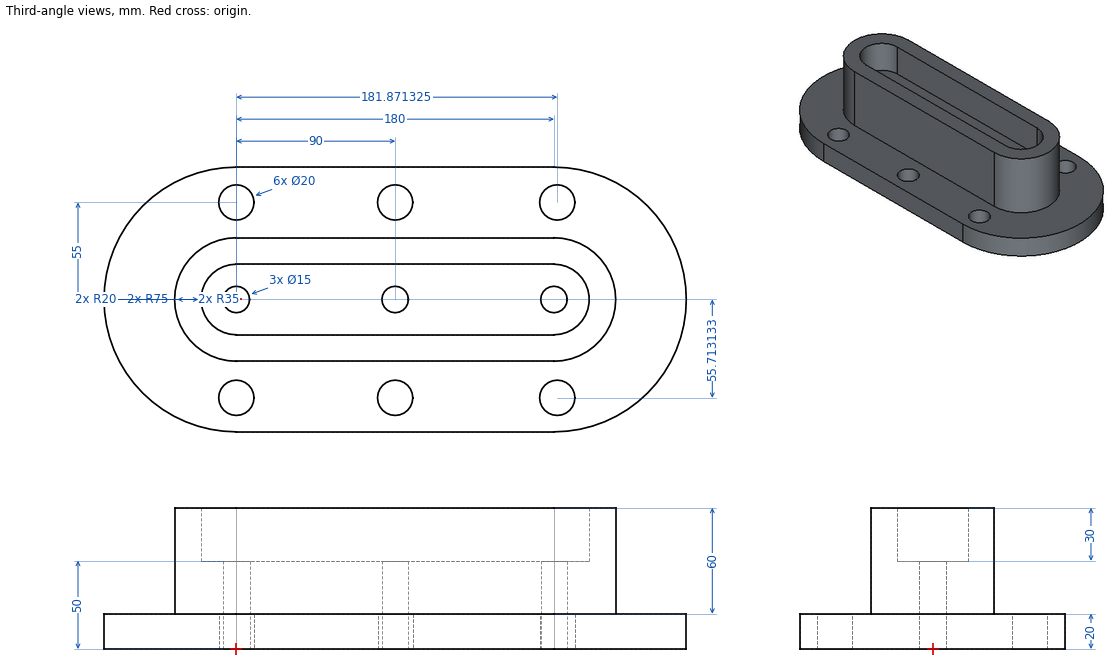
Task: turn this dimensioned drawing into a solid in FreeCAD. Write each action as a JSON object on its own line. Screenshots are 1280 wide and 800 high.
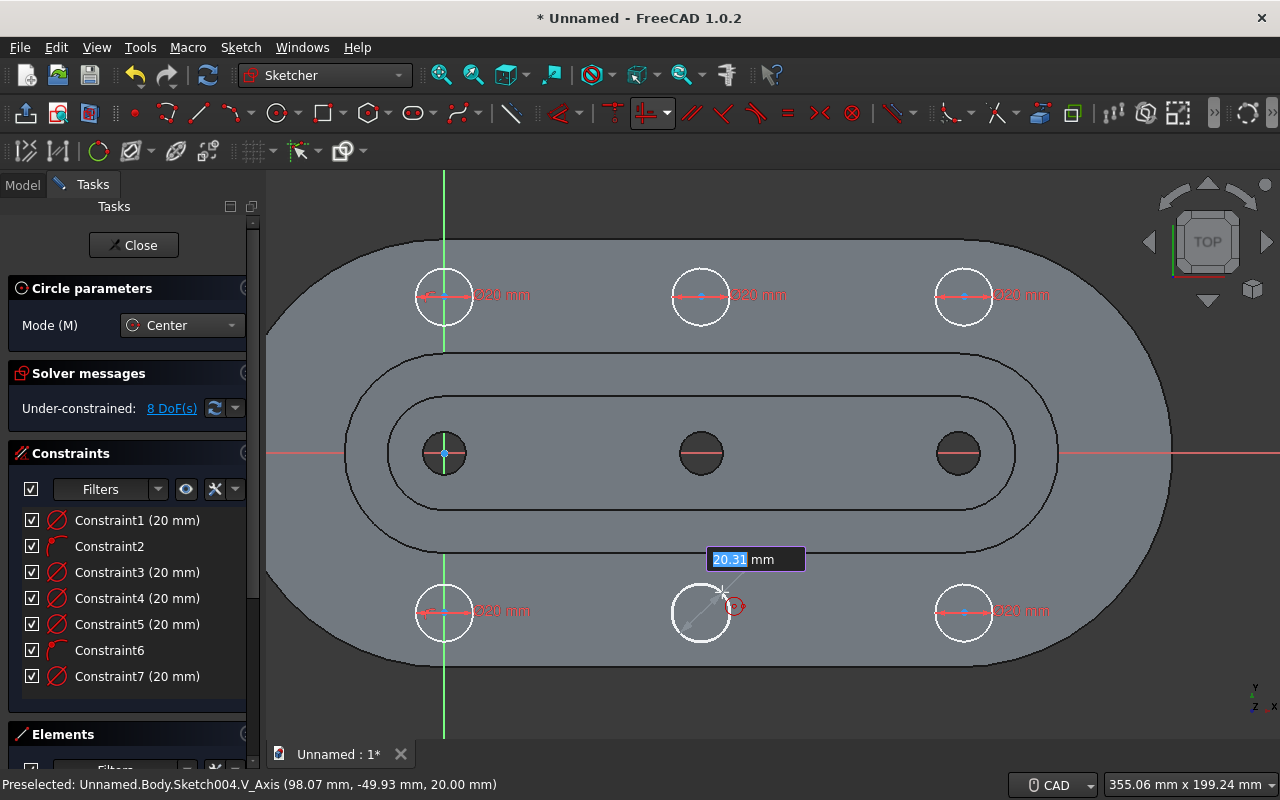
{"action": "type", "text": "20"}
{"action": "key", "text": "Return"}
{"action": "key", "text": "Escape"}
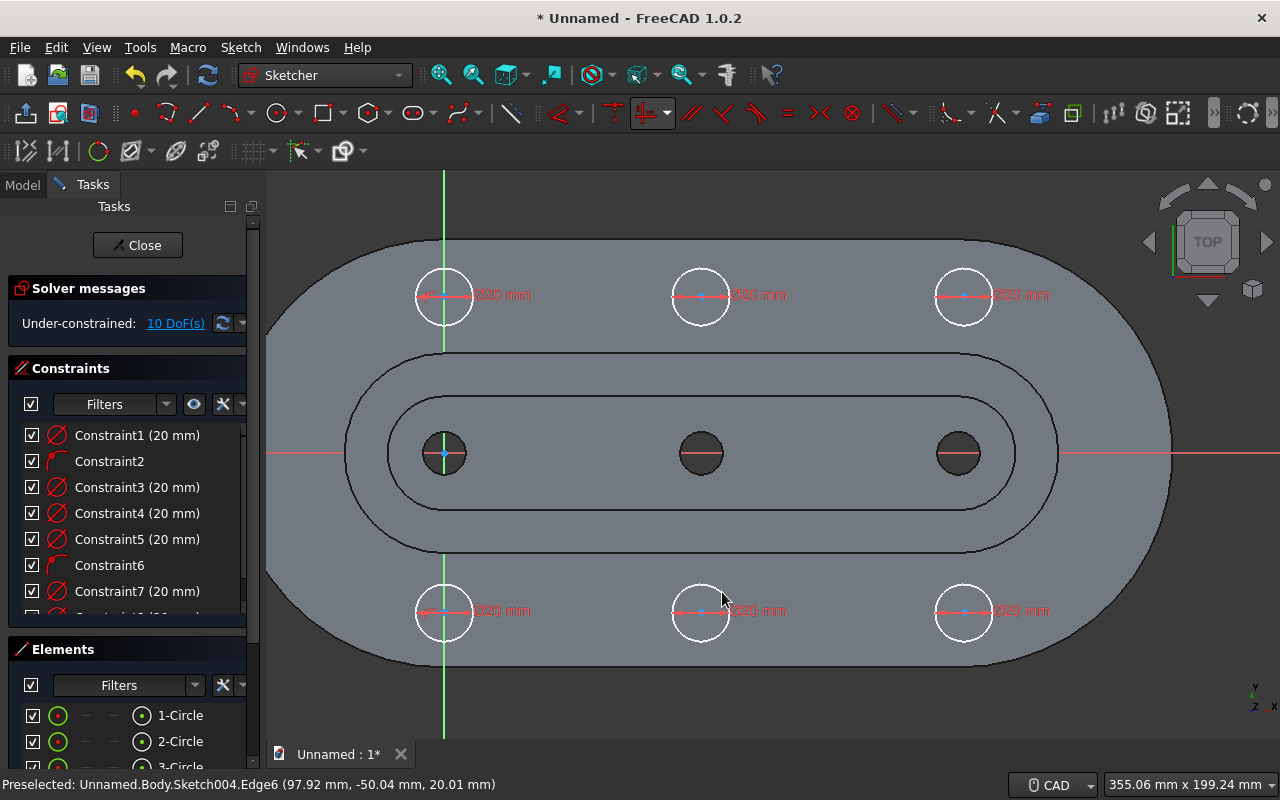
{"action": "left_click", "coordinate": [558, 114]}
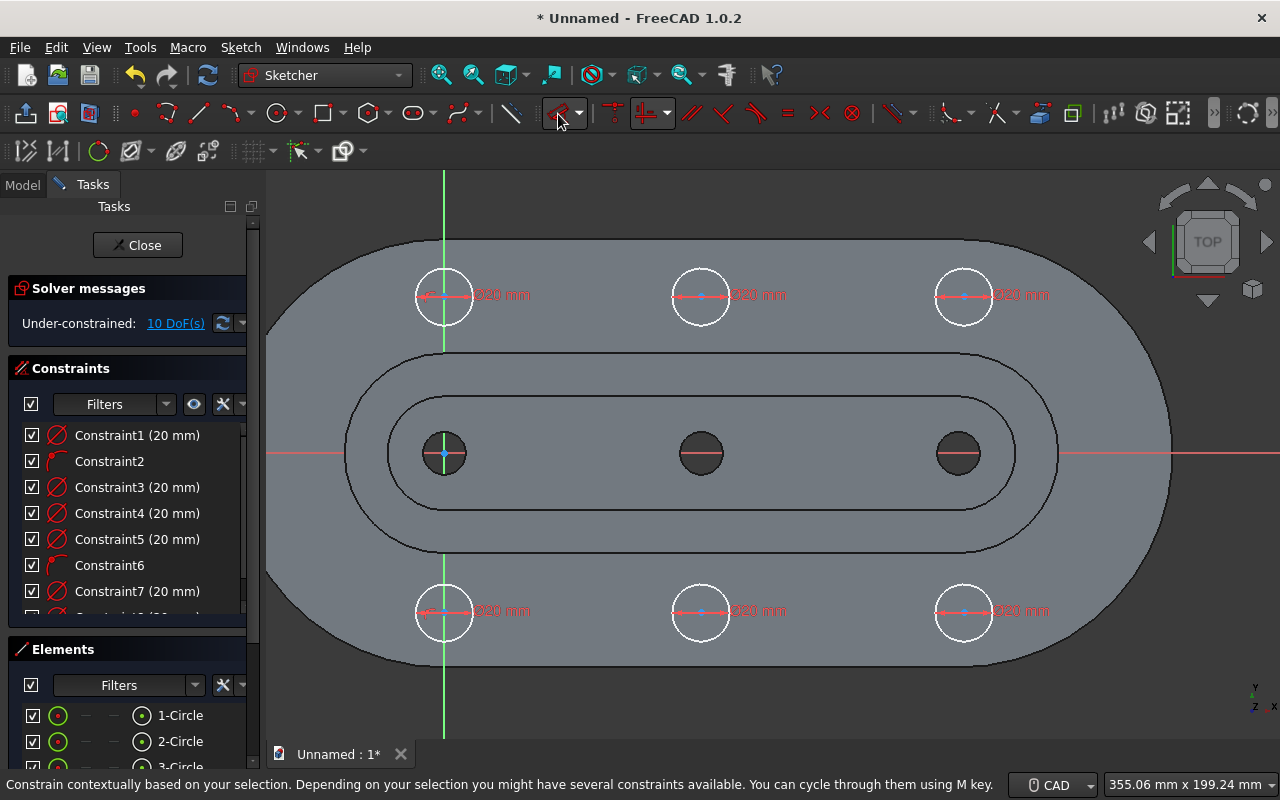
{"action": "left_click", "coordinate": [444, 297]}
{"action": "left_click", "coordinate": [410, 375]}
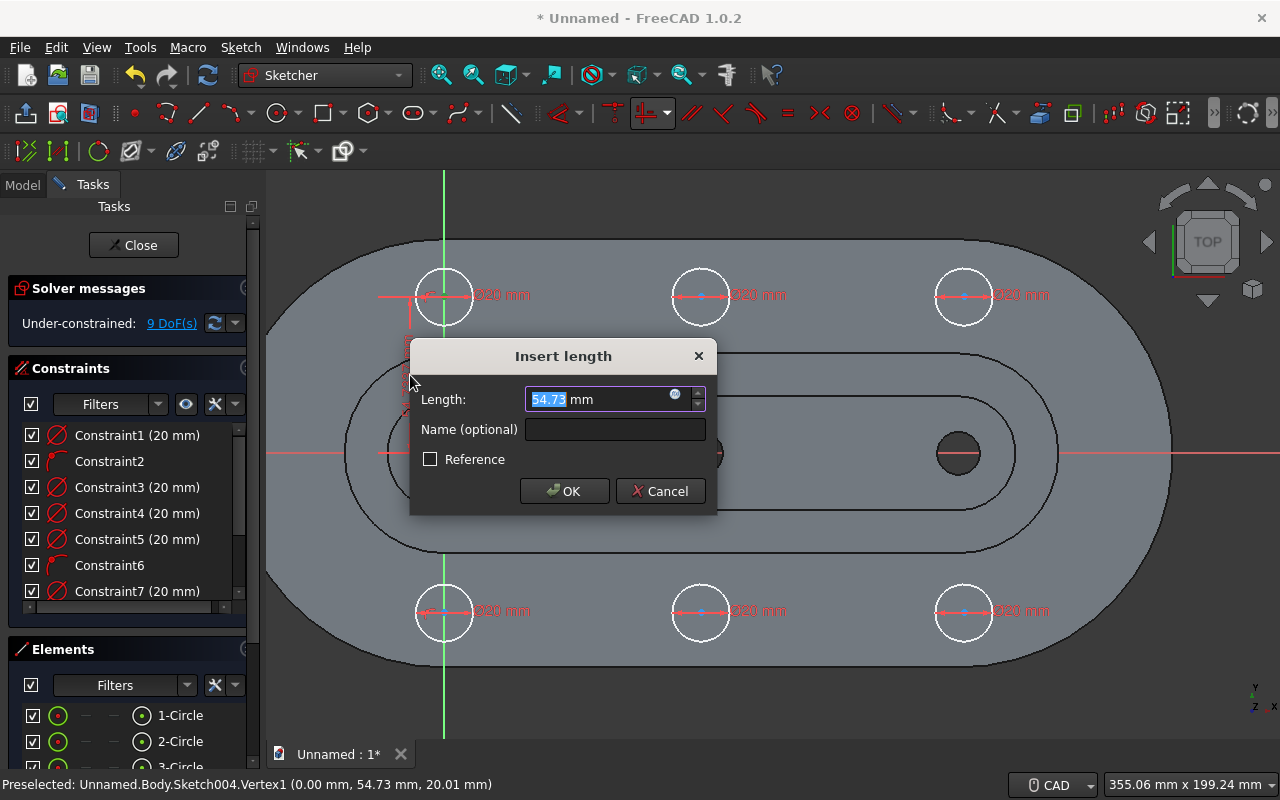
{"action": "type", "text": "55"}
{"action": "key", "text": "Return"}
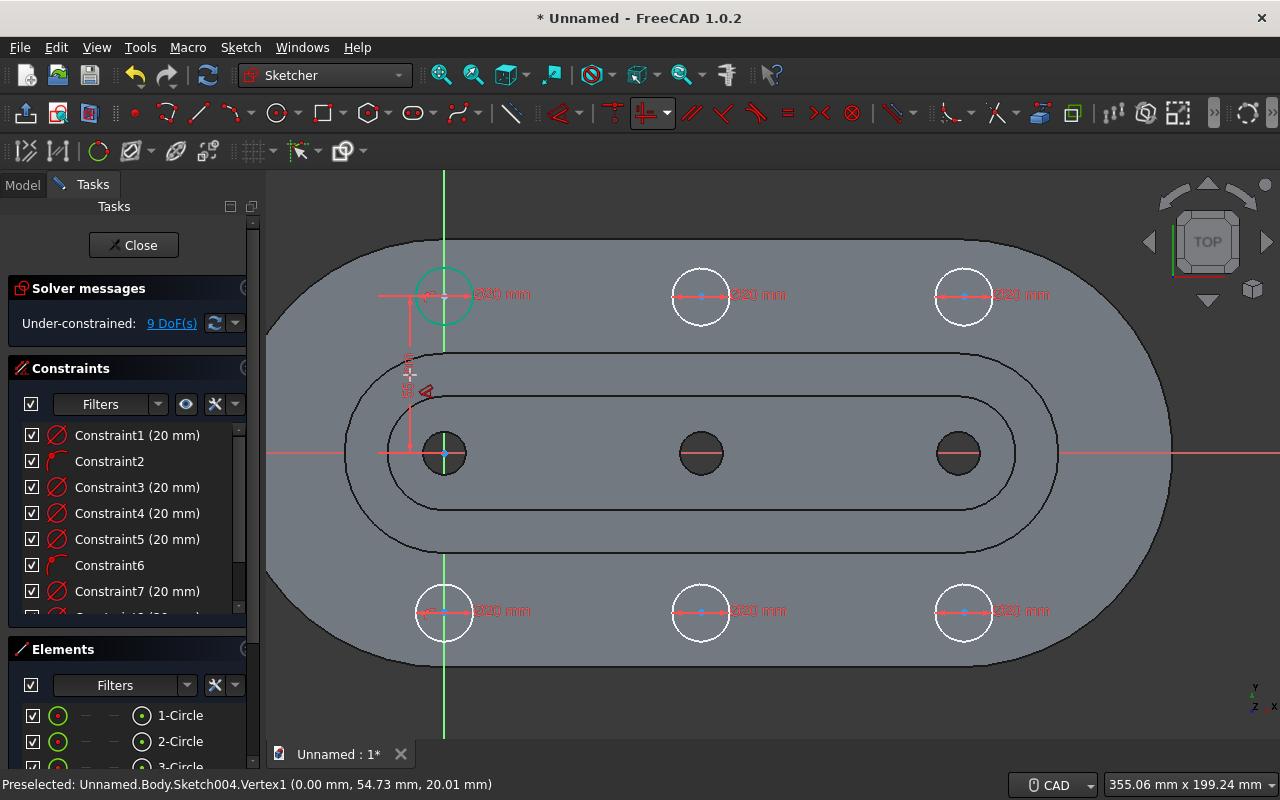
{"action": "left_click", "coordinate": [964, 297]}
{"action": "left_click", "coordinate": [998, 375]}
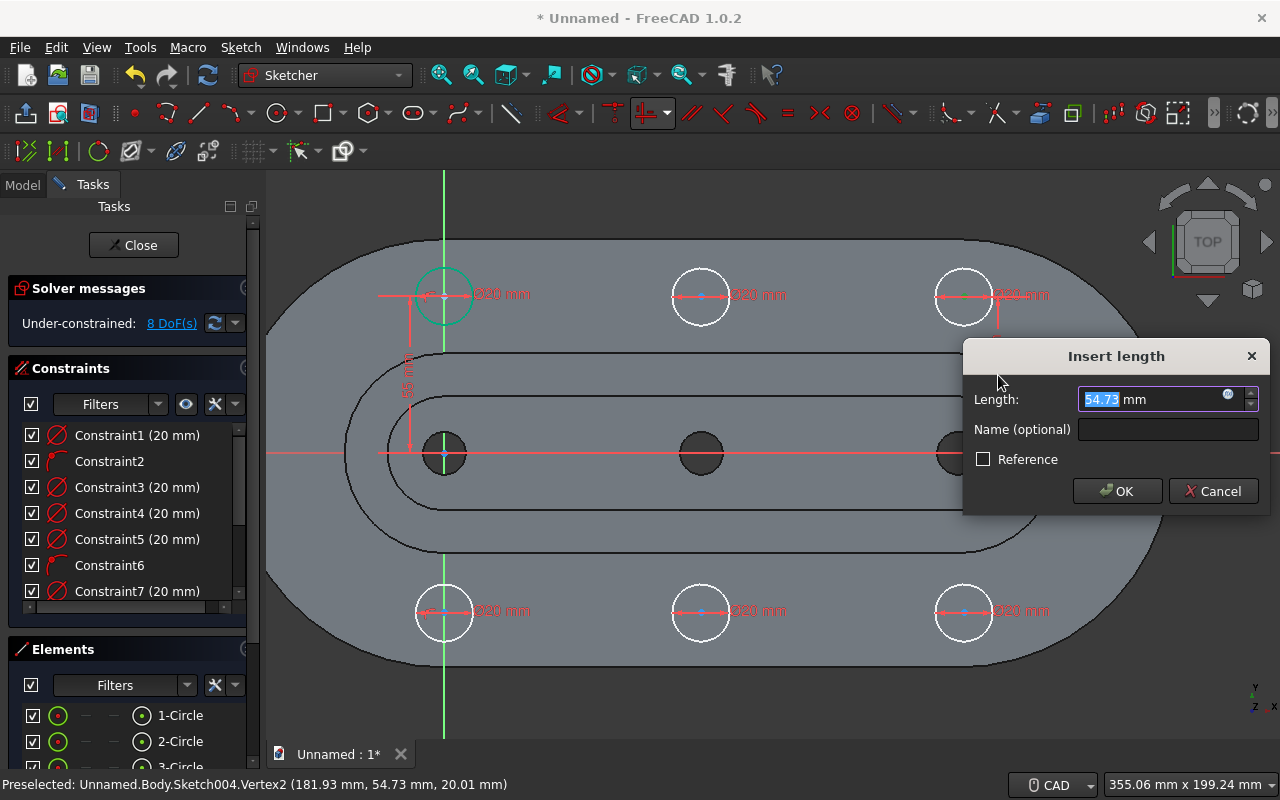
{"action": "type", "text": "55"}
{"action": "key", "text": "Return"}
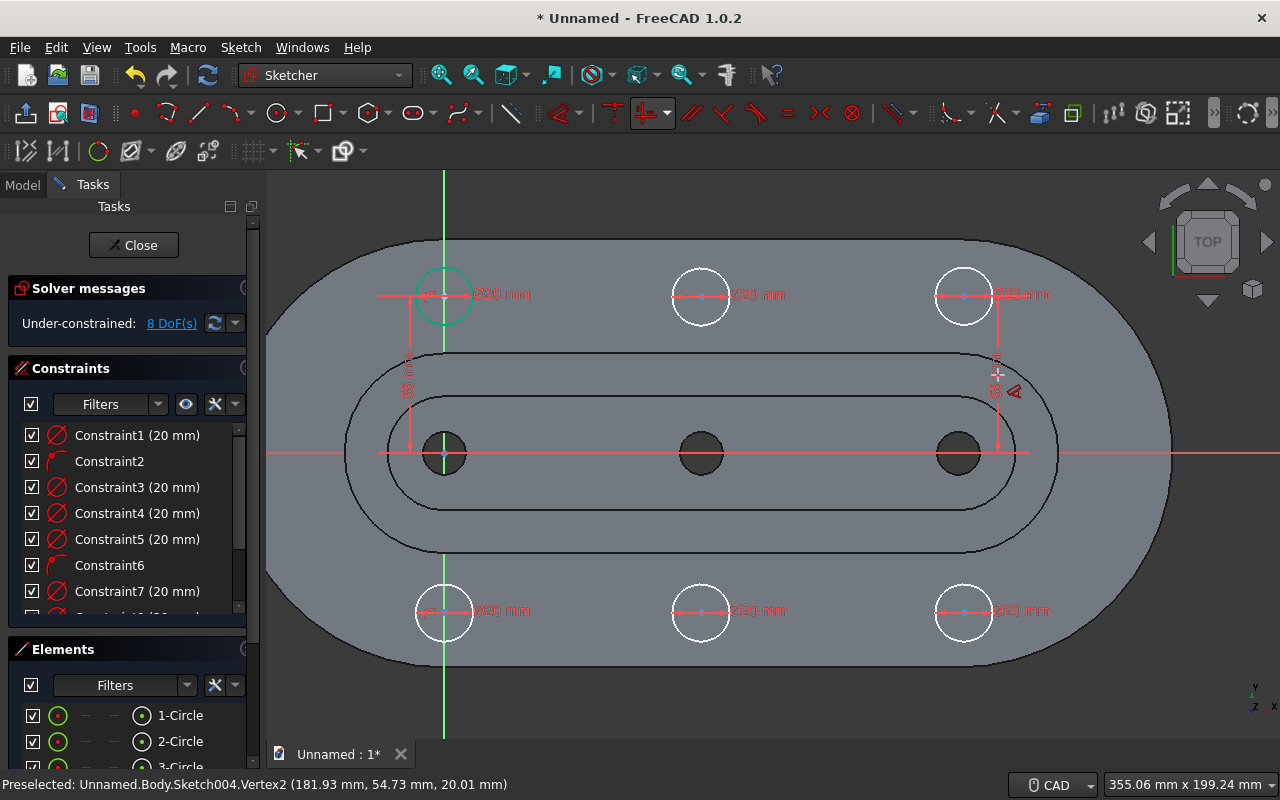
{"action": "left_click", "coordinate": [701, 297]}
{"action": "left_click", "coordinate": [573, 263]}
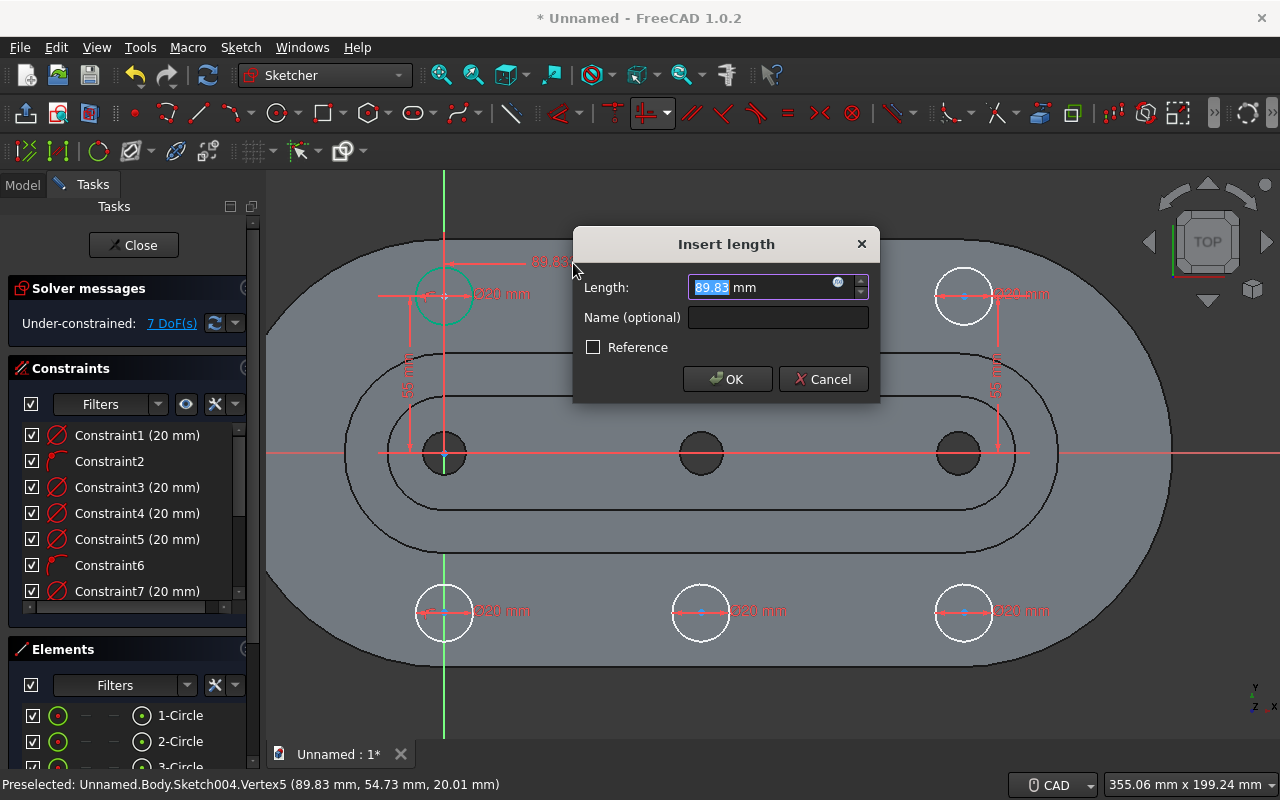
{"action": "type", "text": "90"}
{"action": "key", "text": "Return"}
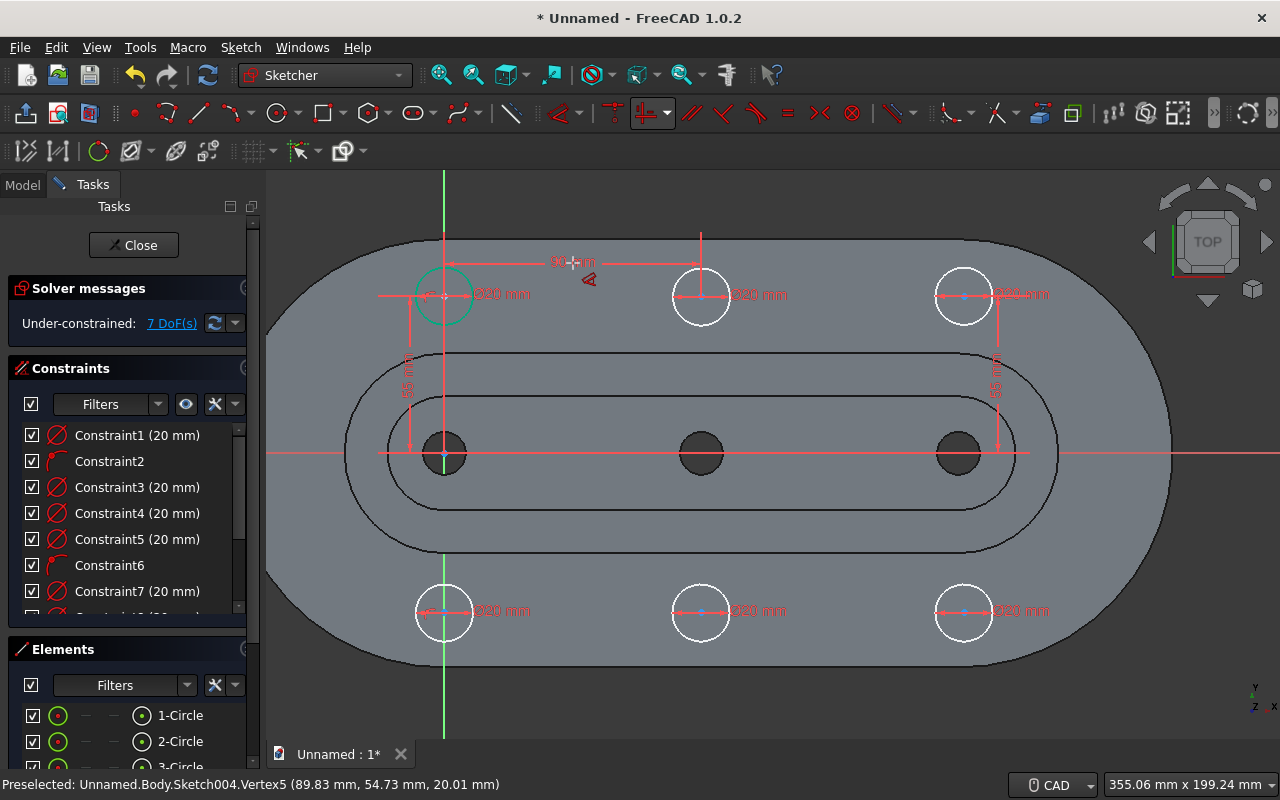
{"action": "left_click", "coordinate": [701, 297]}
{"action": "left_click", "coordinate": [410, 339]}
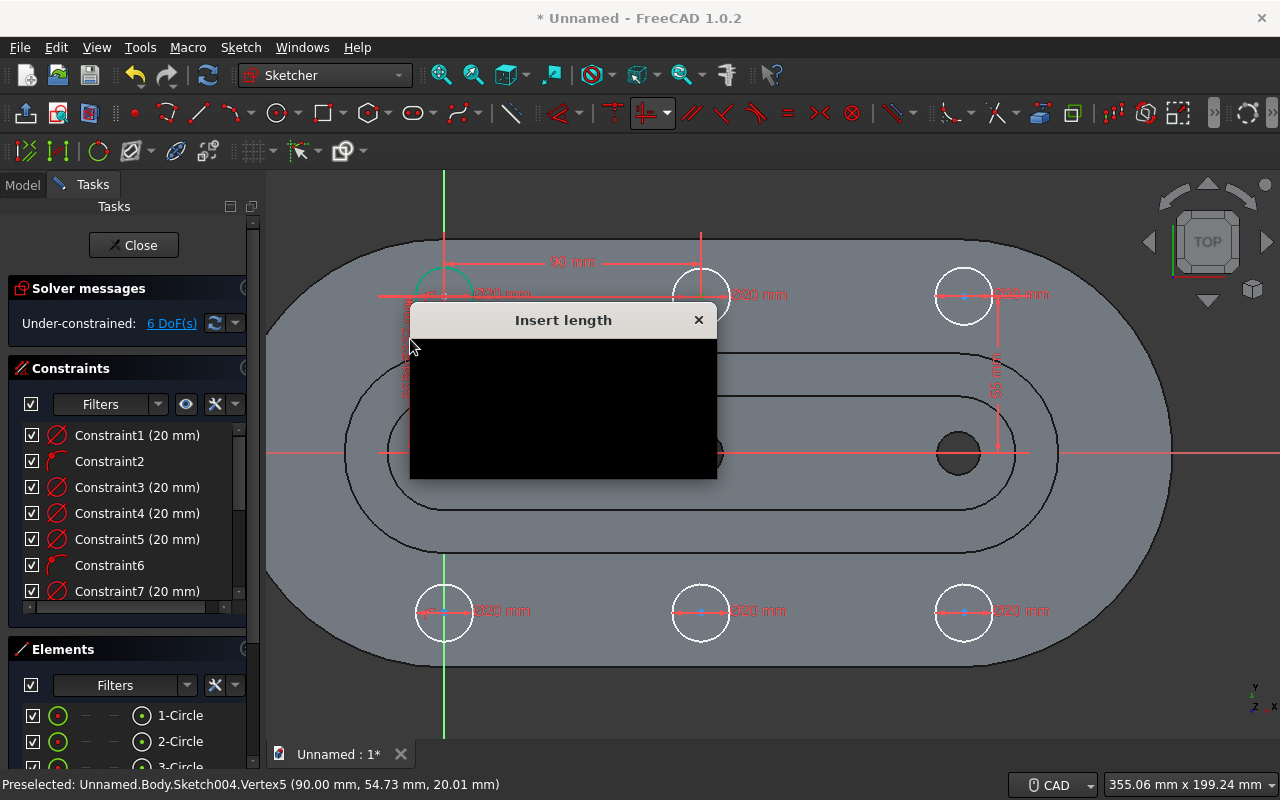
{"action": "type", "text": "55"}
{"action": "key", "text": "Return"}